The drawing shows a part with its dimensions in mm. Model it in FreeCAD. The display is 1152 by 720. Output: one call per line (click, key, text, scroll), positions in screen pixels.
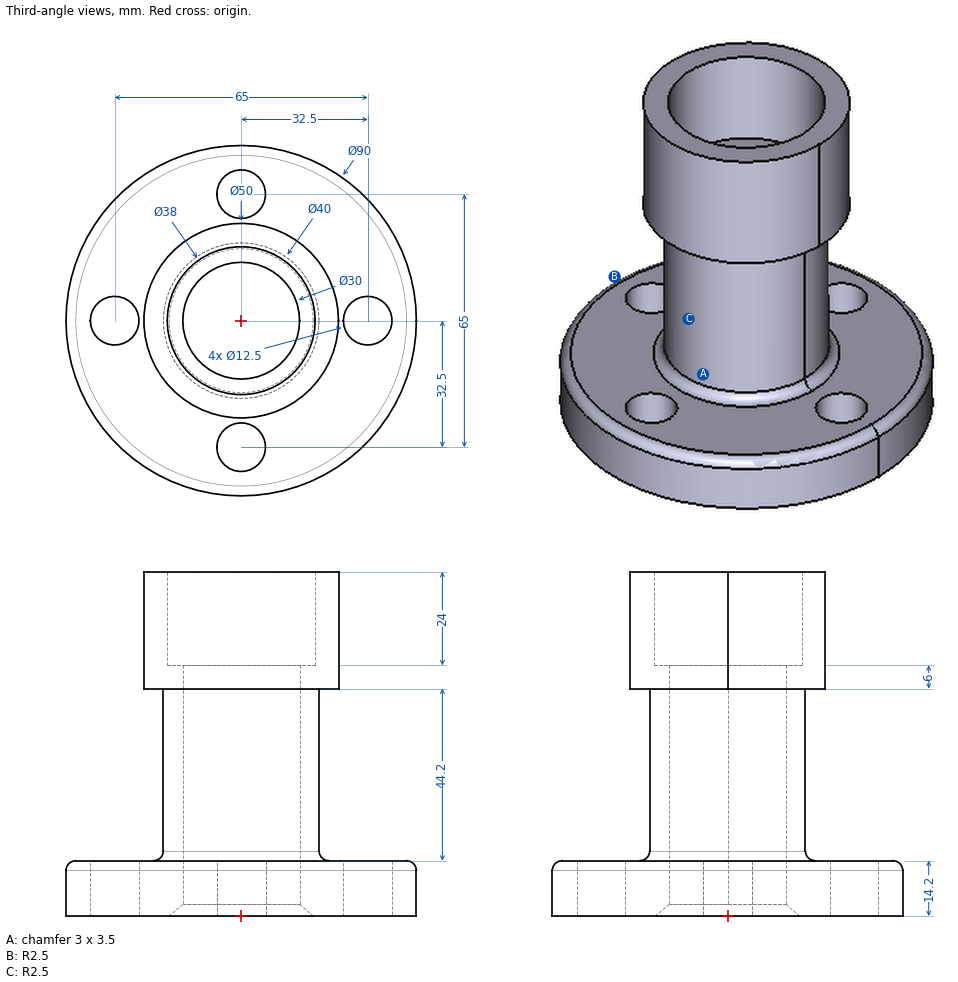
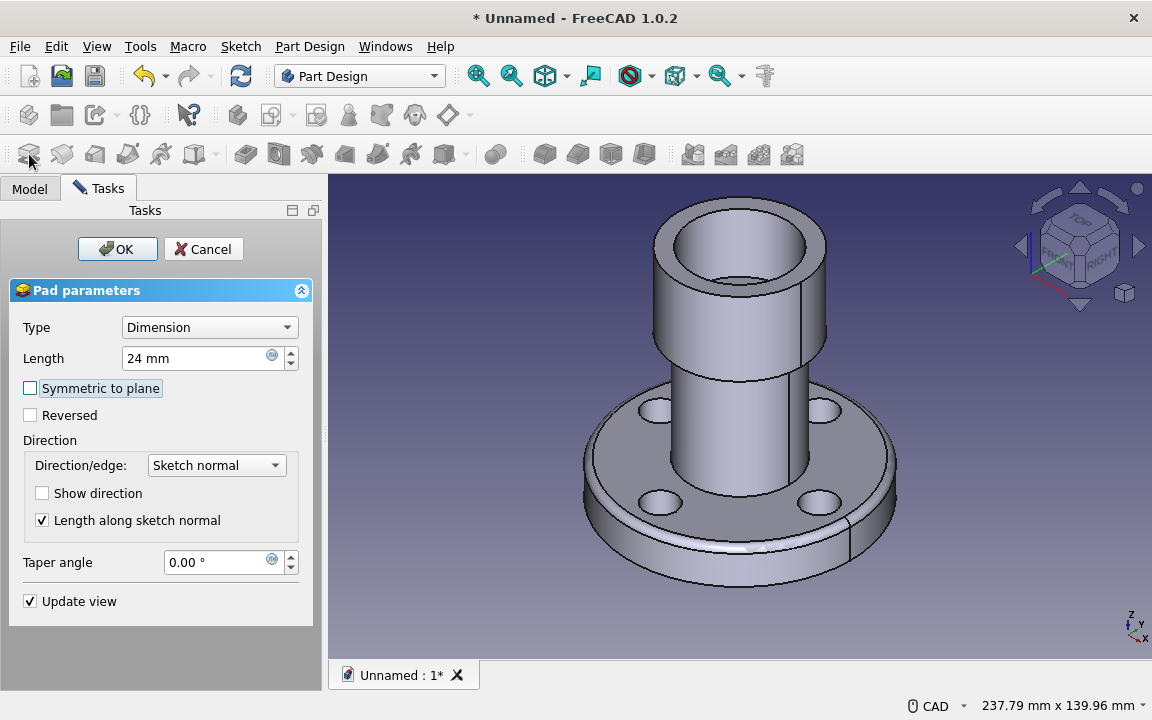
click(118, 249)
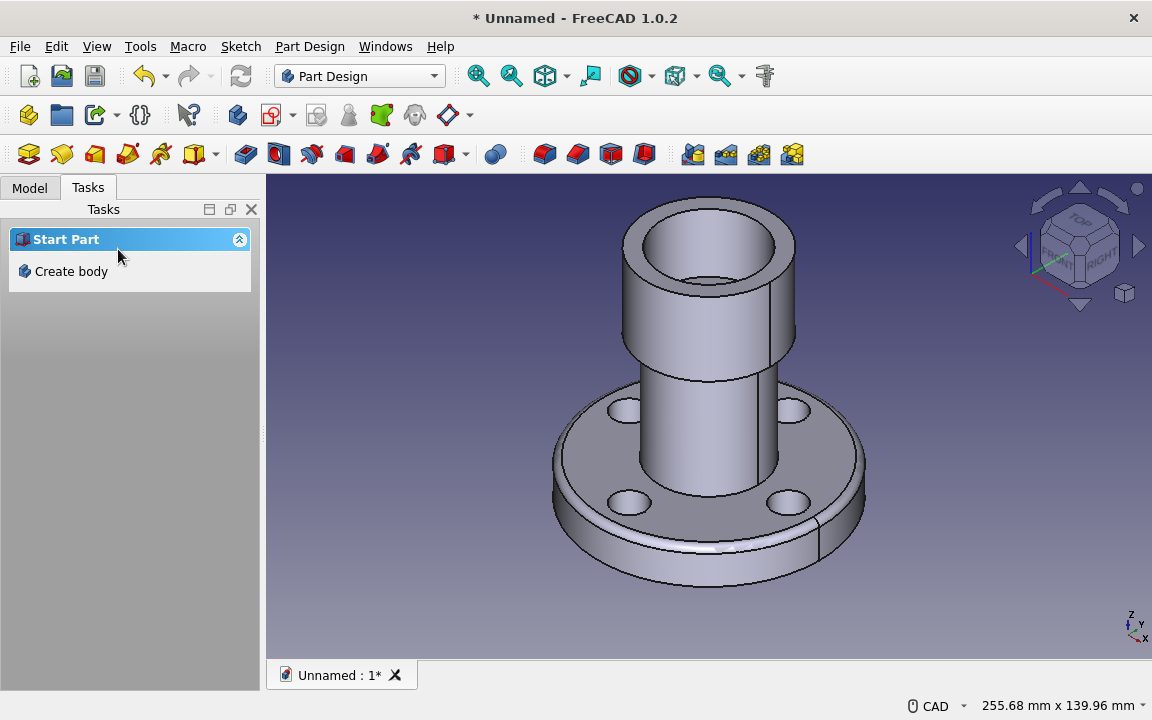
click(479, 76)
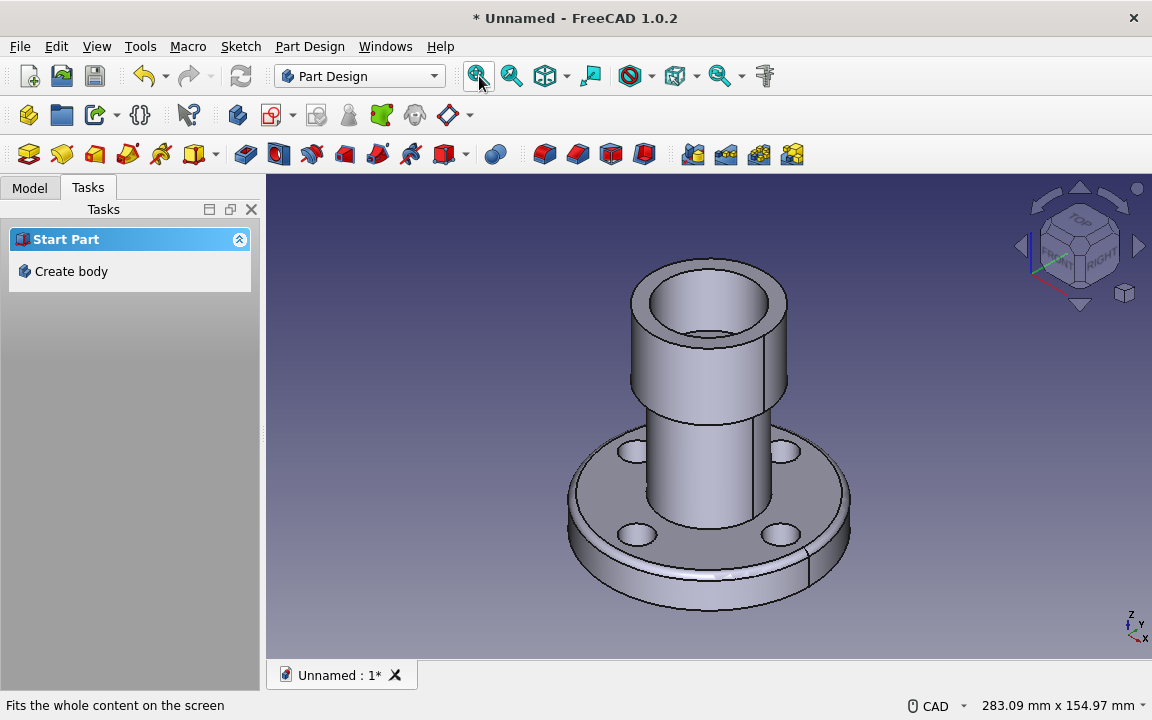
key(2)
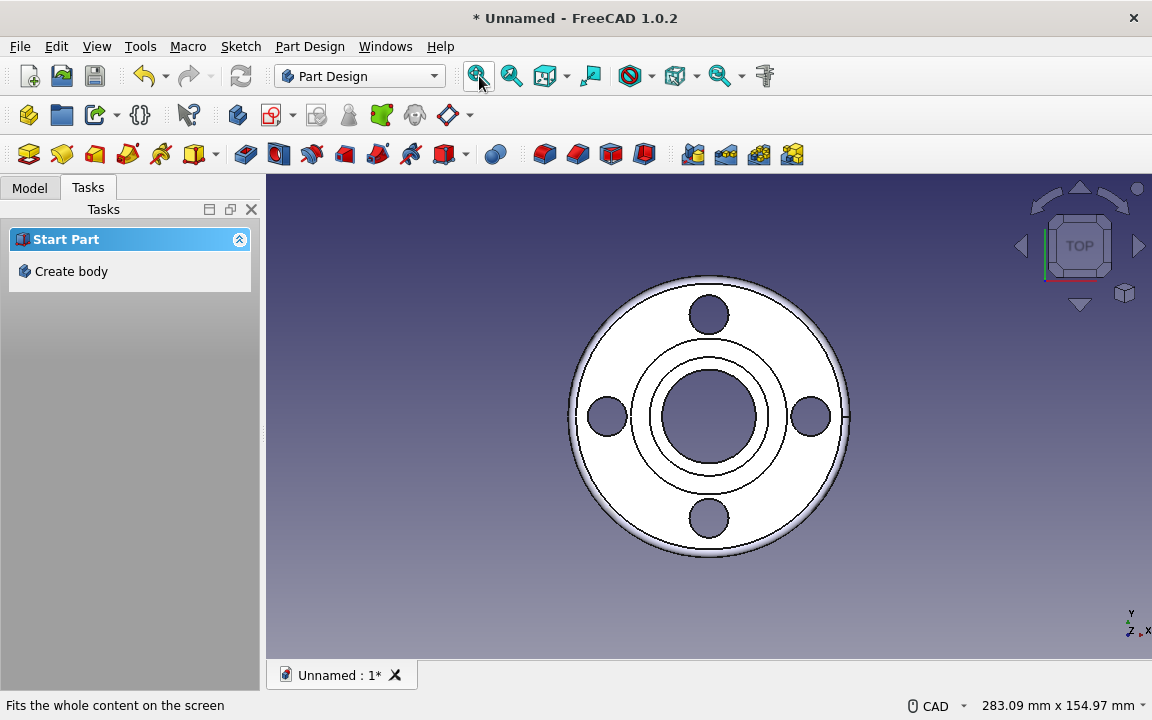
key(0)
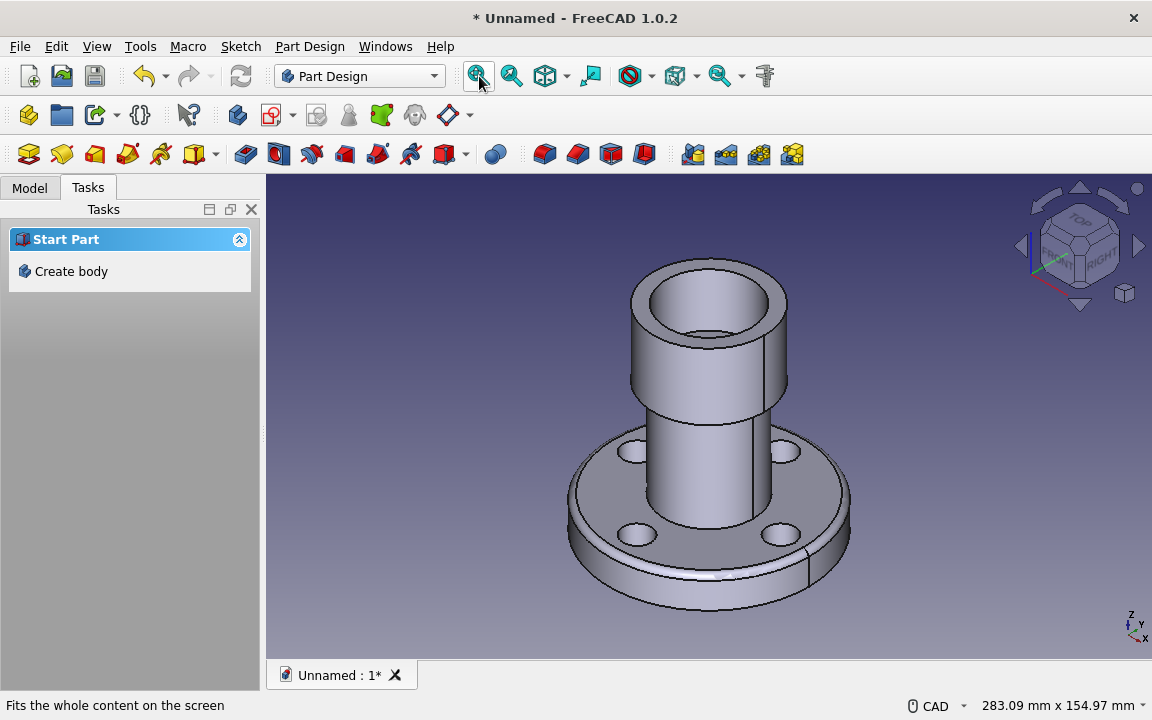
key(1)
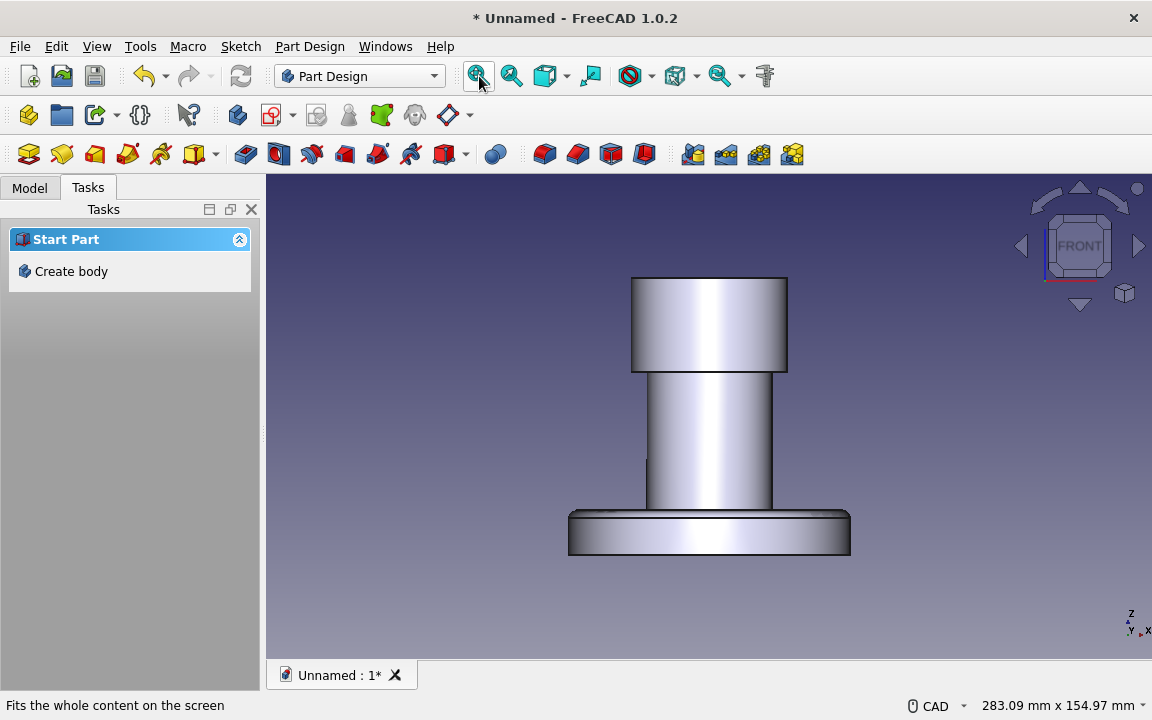
key(3)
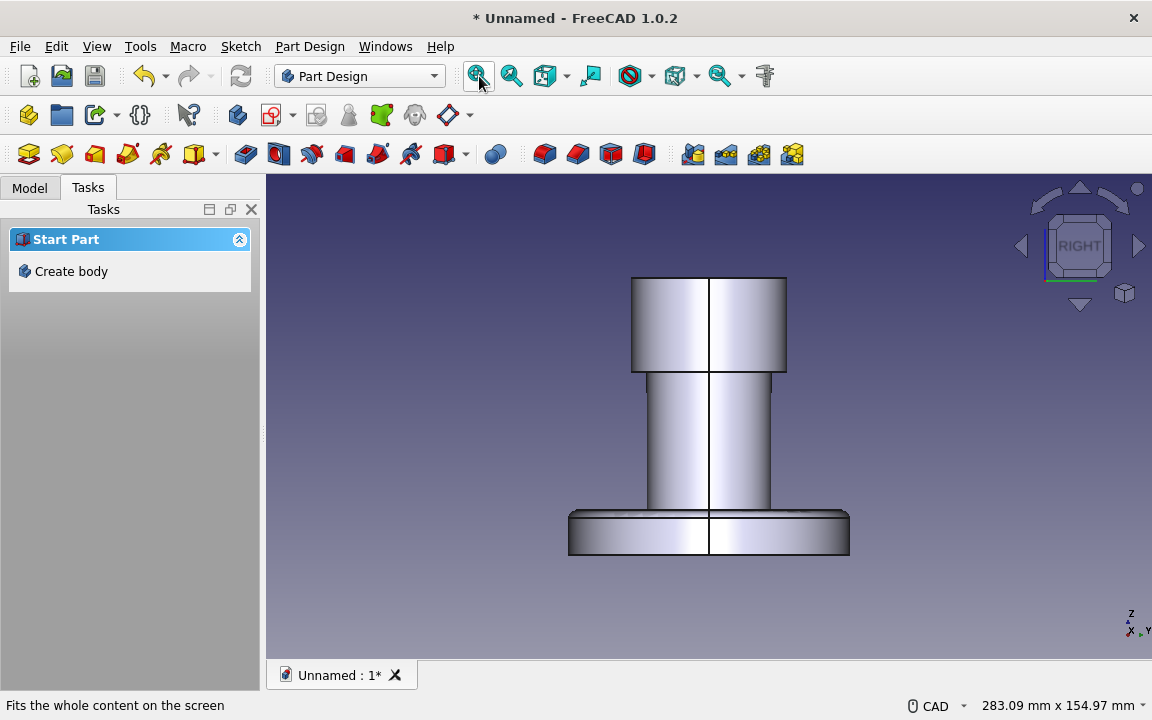
key(5)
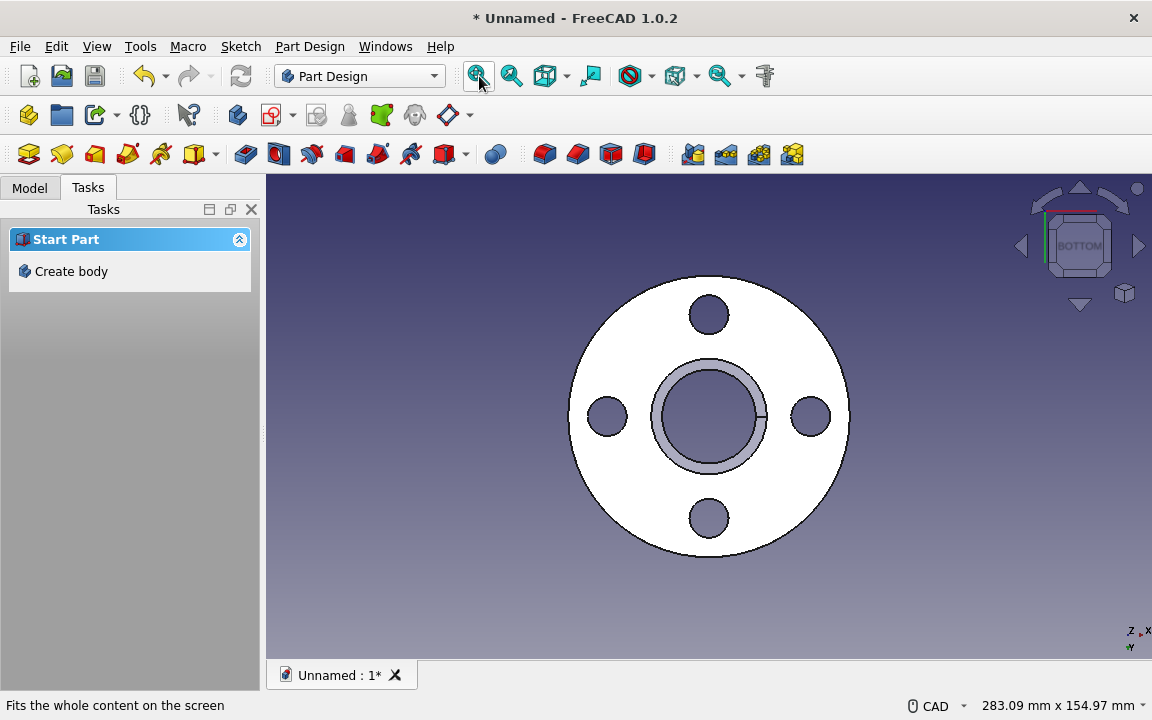
key(4)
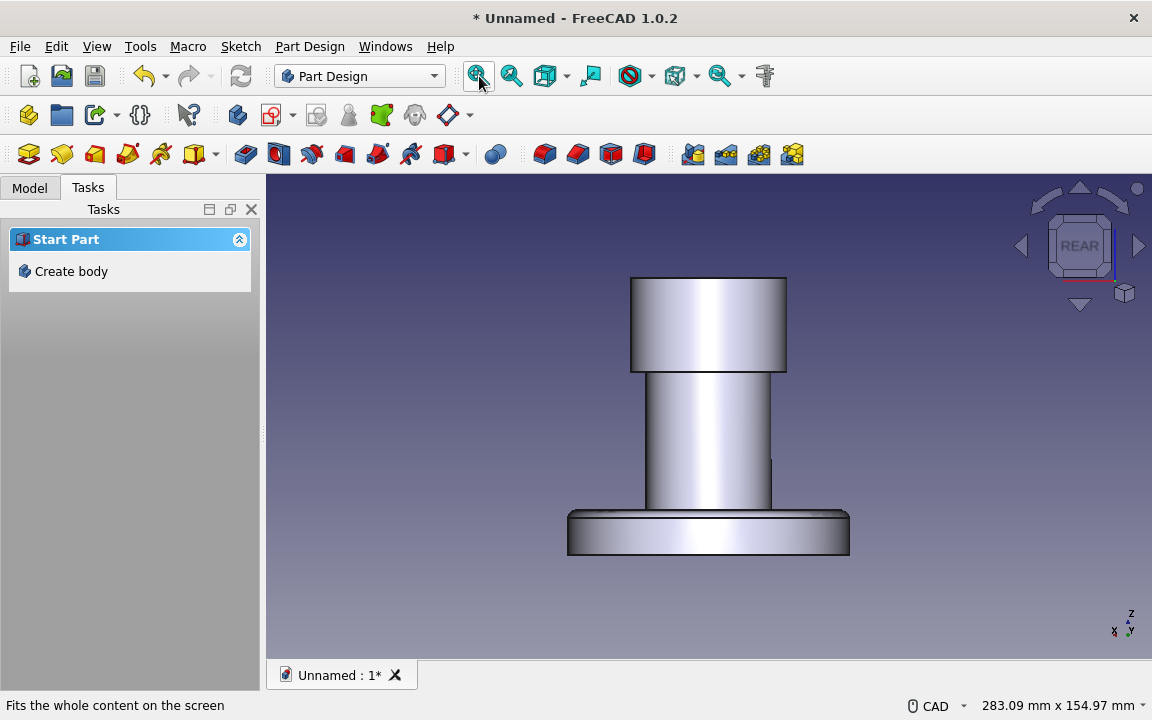
key(6)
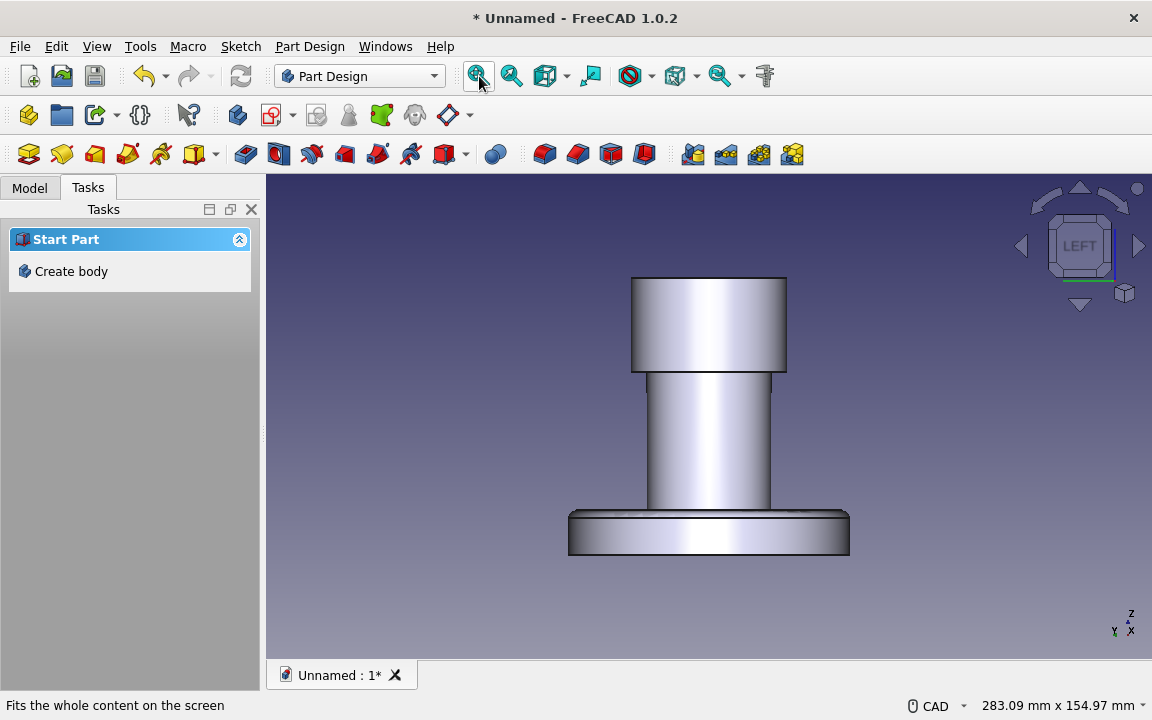
key(v)
key(3)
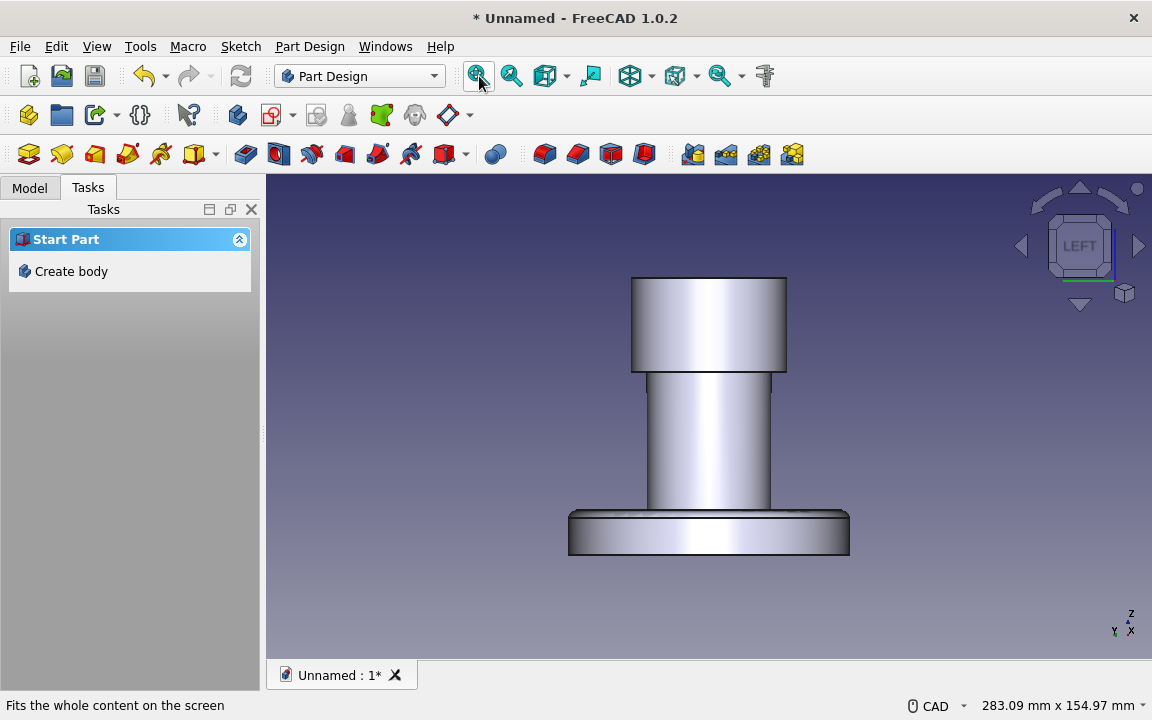
key(0)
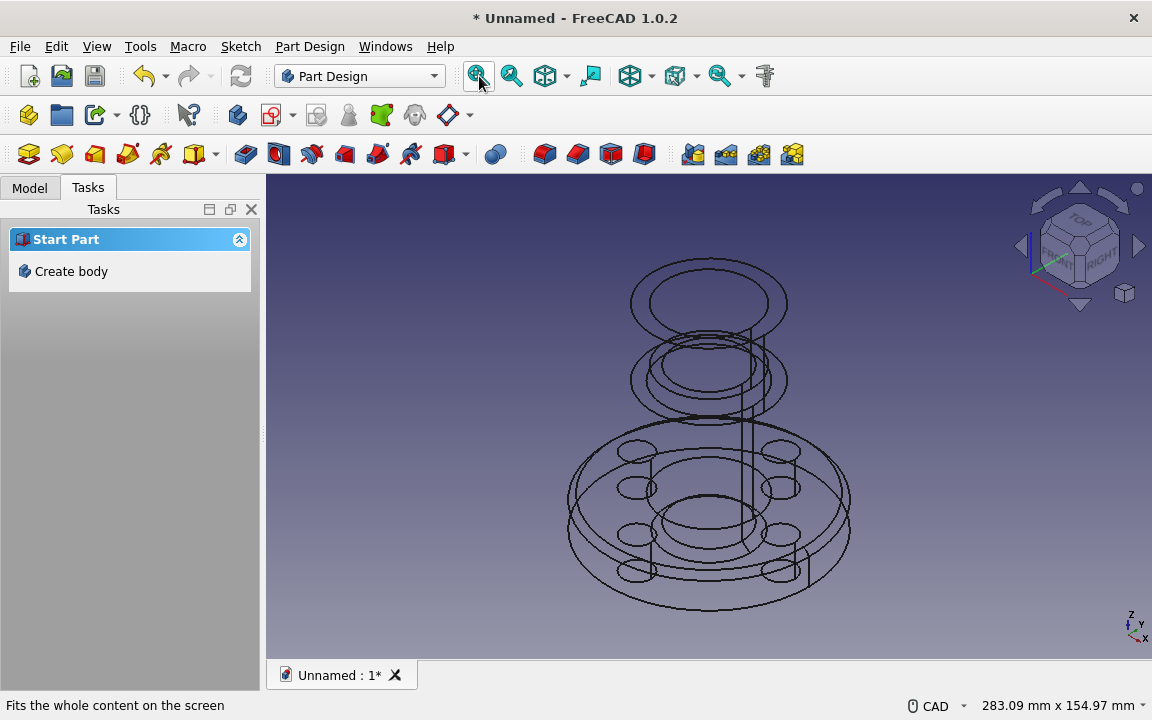
click(665, 467)